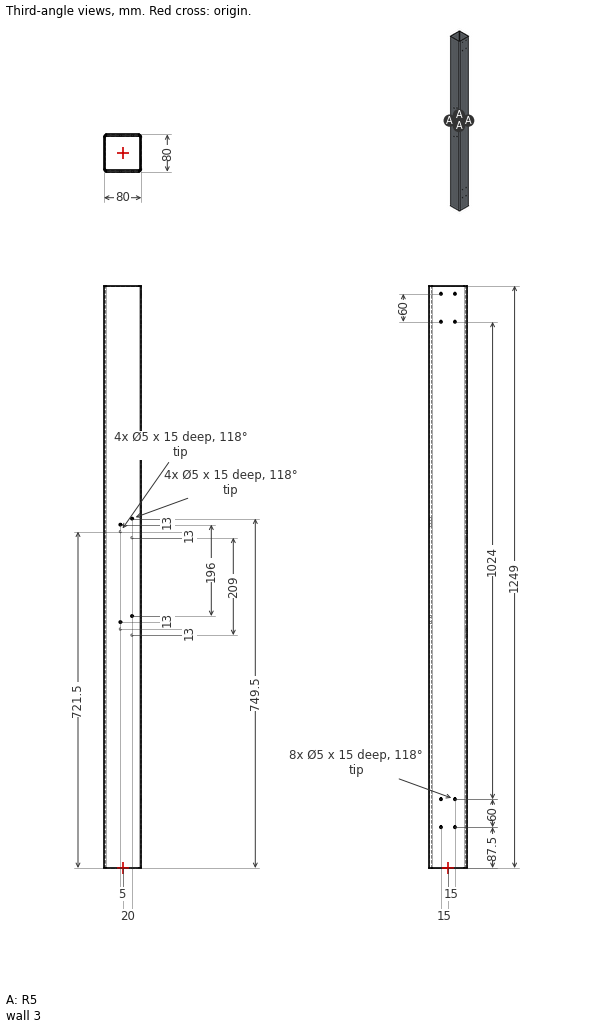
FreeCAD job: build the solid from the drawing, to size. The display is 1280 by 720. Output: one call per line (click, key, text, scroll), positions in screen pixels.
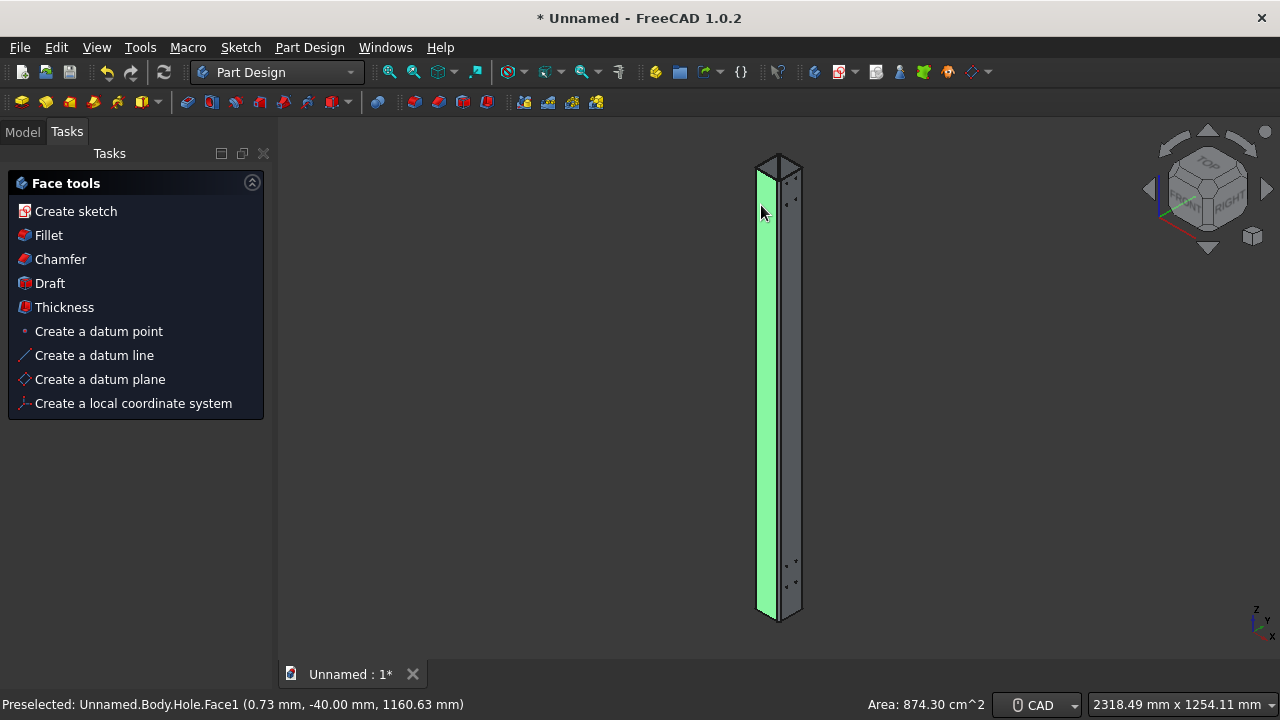
click(840, 72)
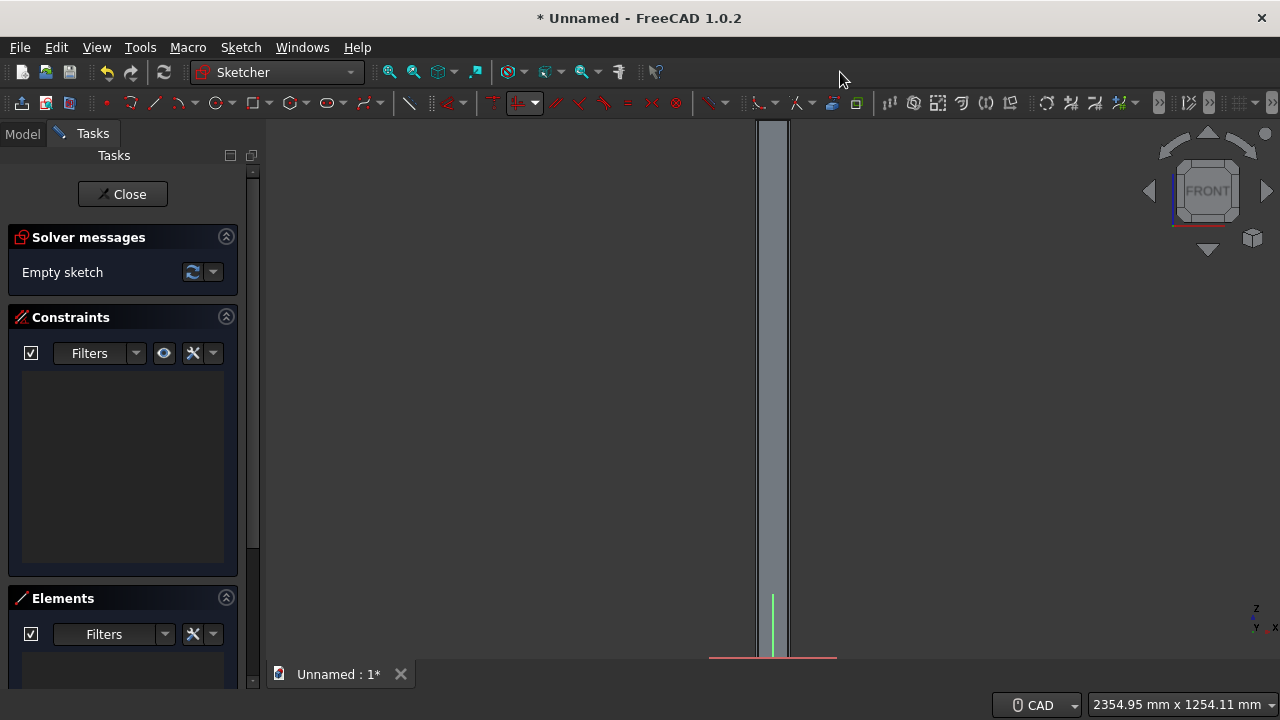
scroll(807, 380, up, 6)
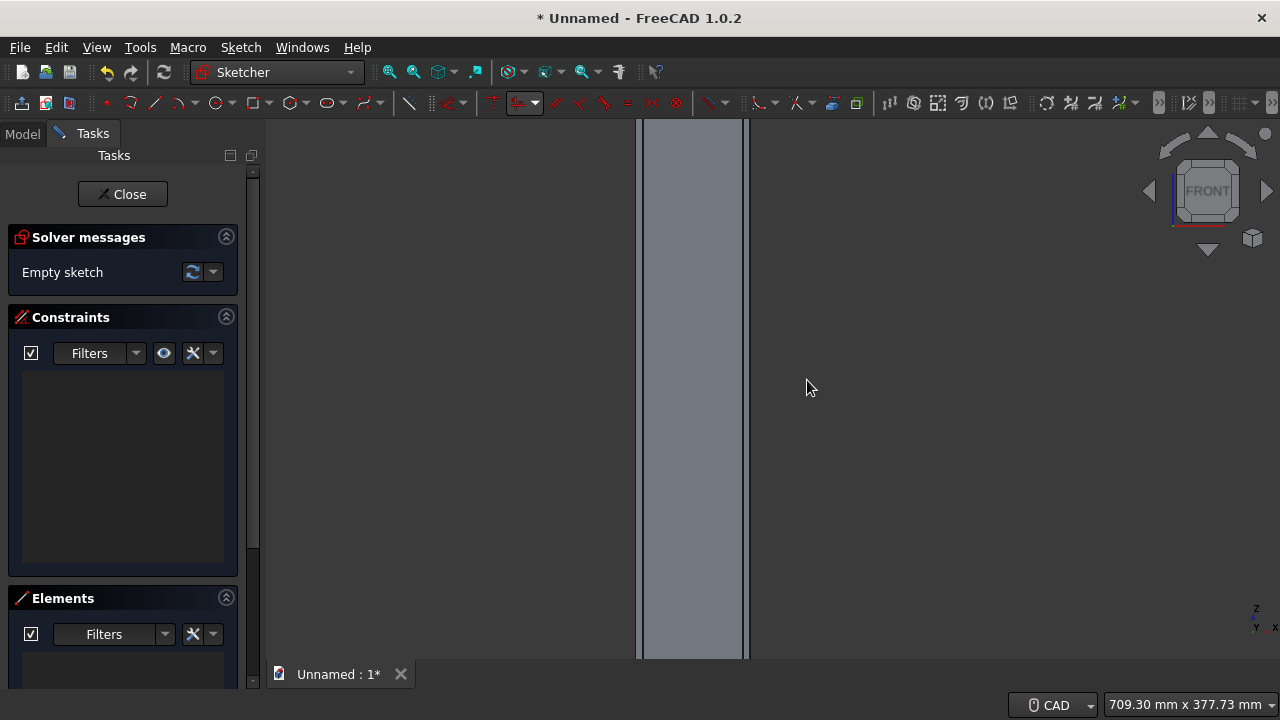
click(216, 104)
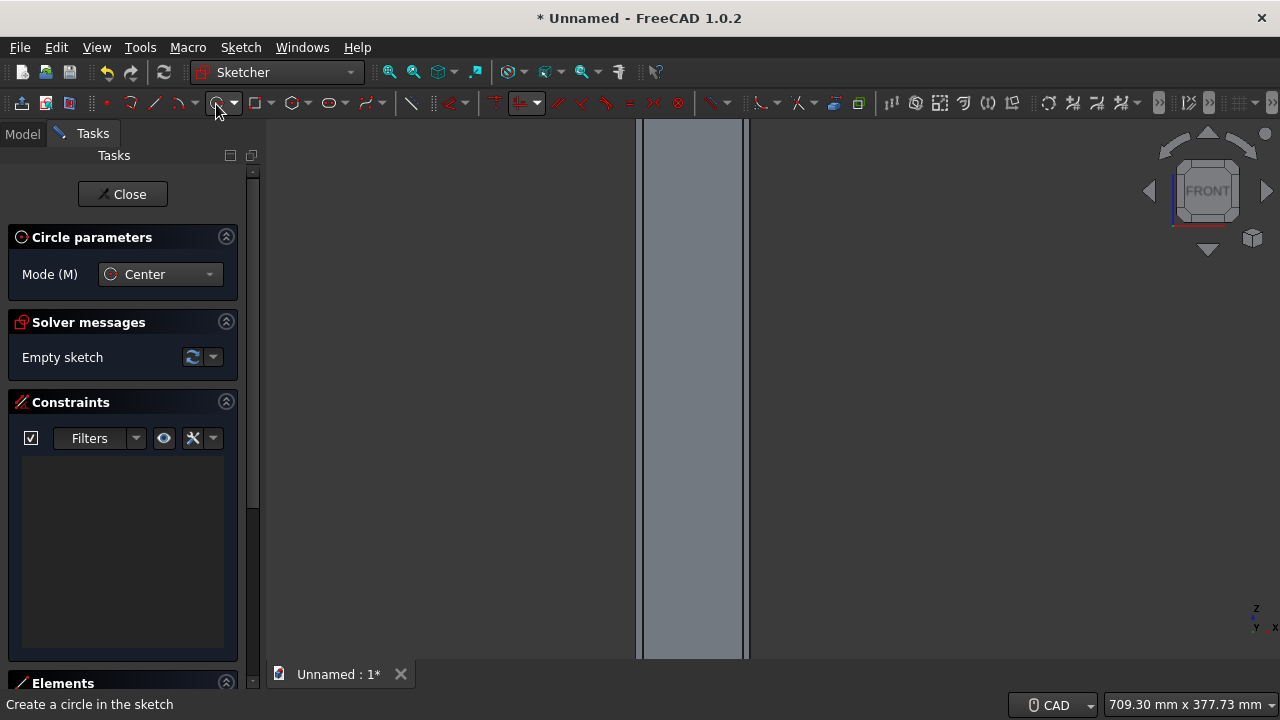
scroll(721, 230, up, 10)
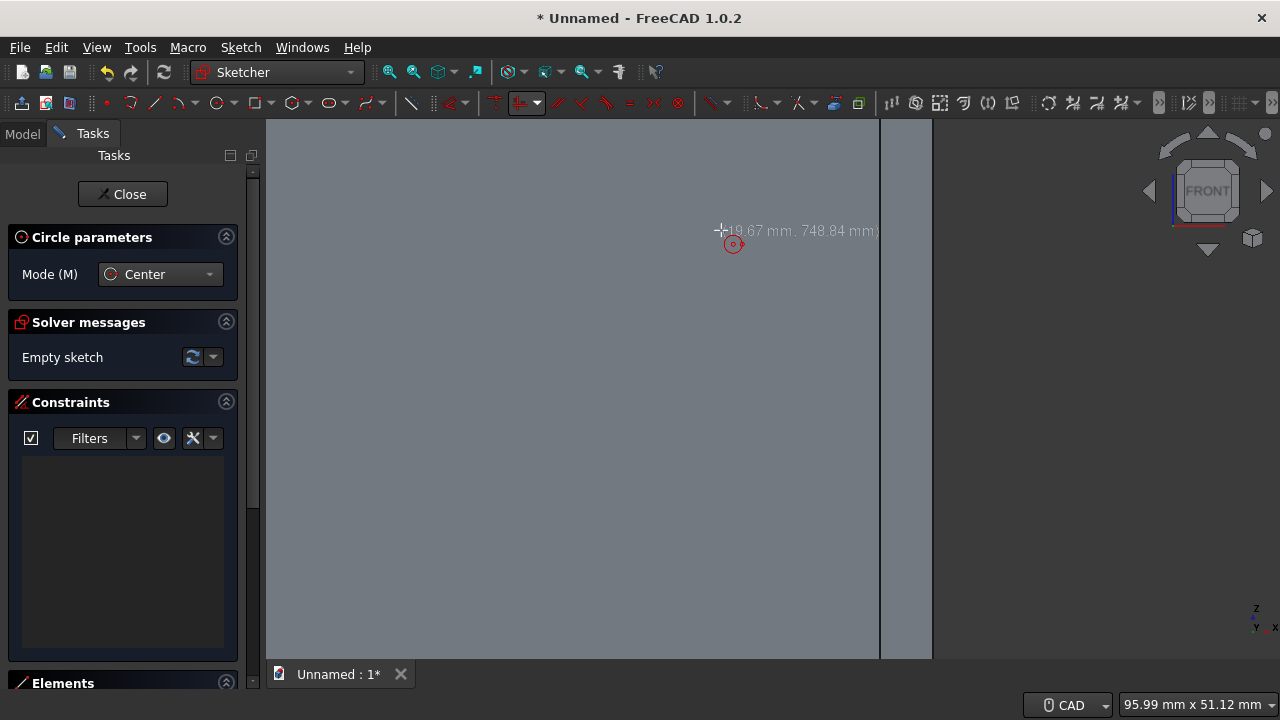
scroll(722, 231, down, 10)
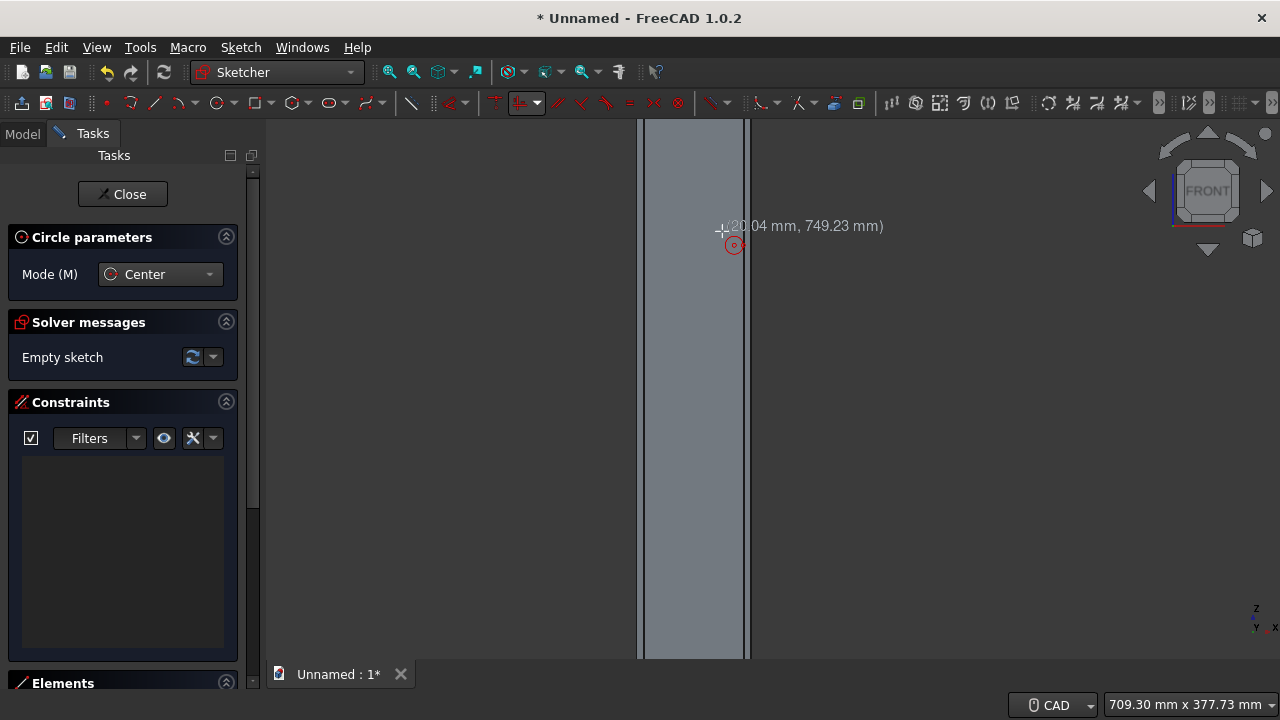
click(722, 231)
move(725, 228)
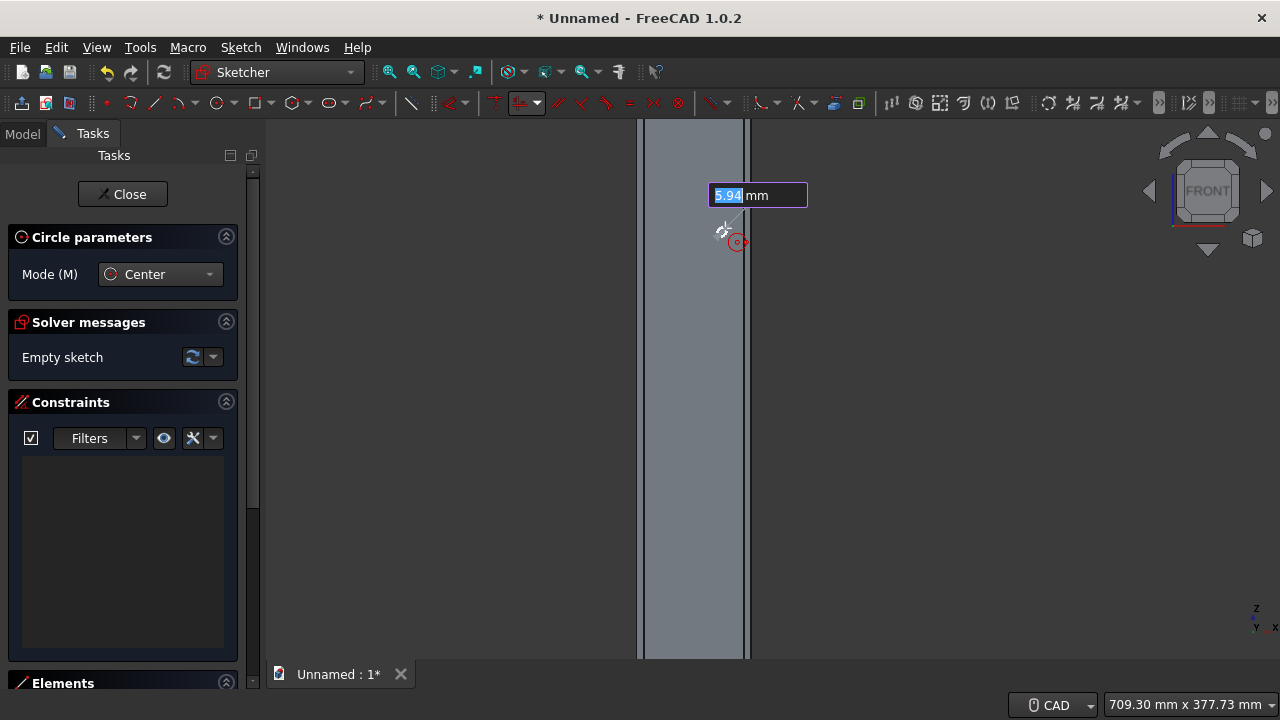
text(5)
key(Return)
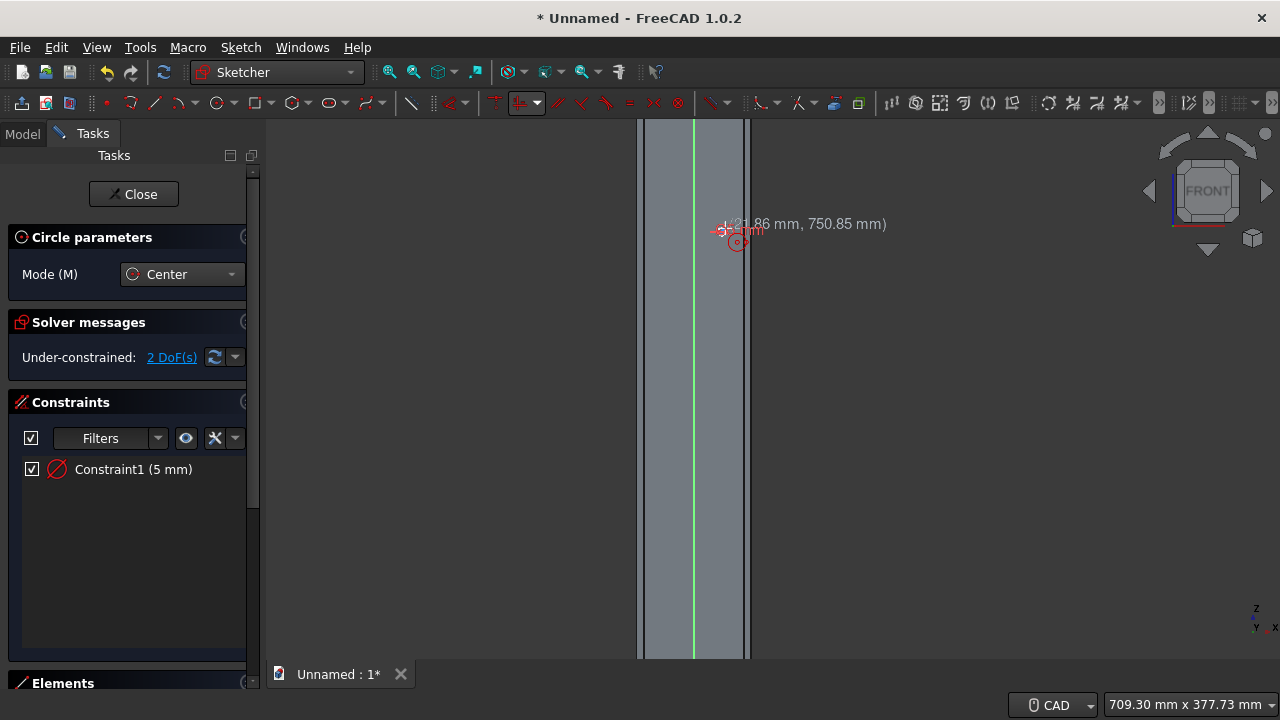
scroll(687, 250, up, 10)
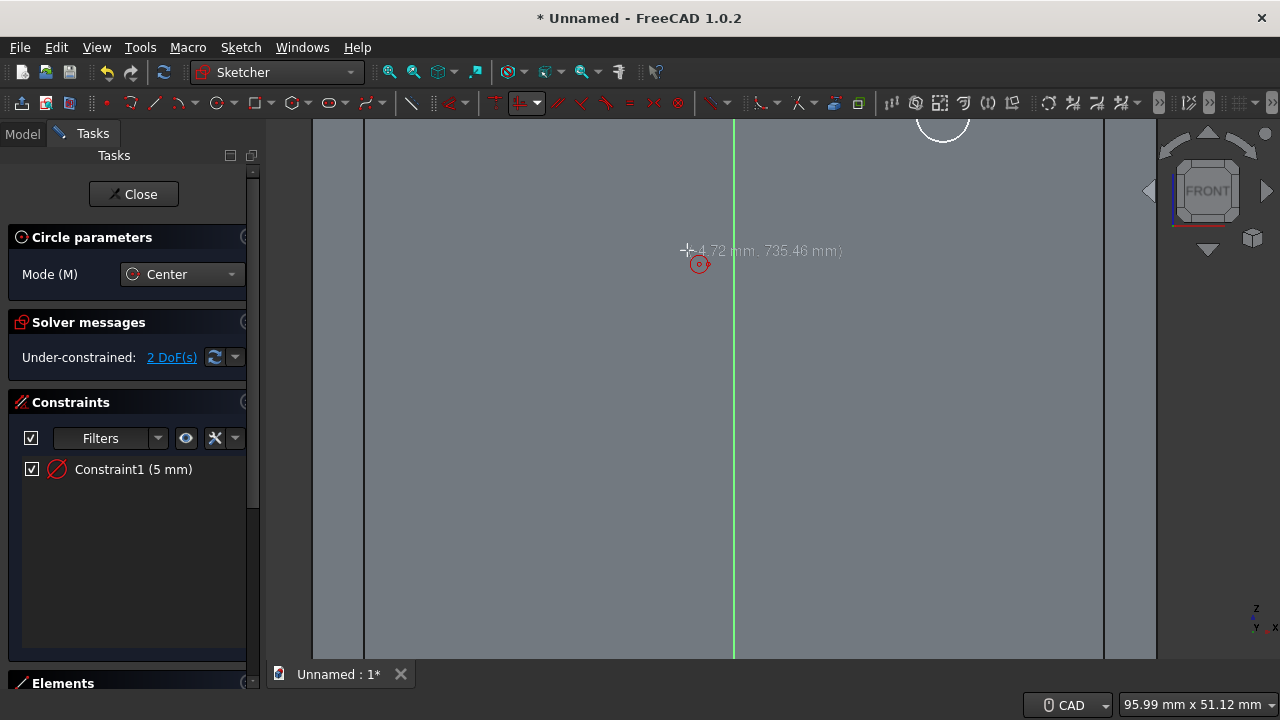
scroll(687, 250, down, 10)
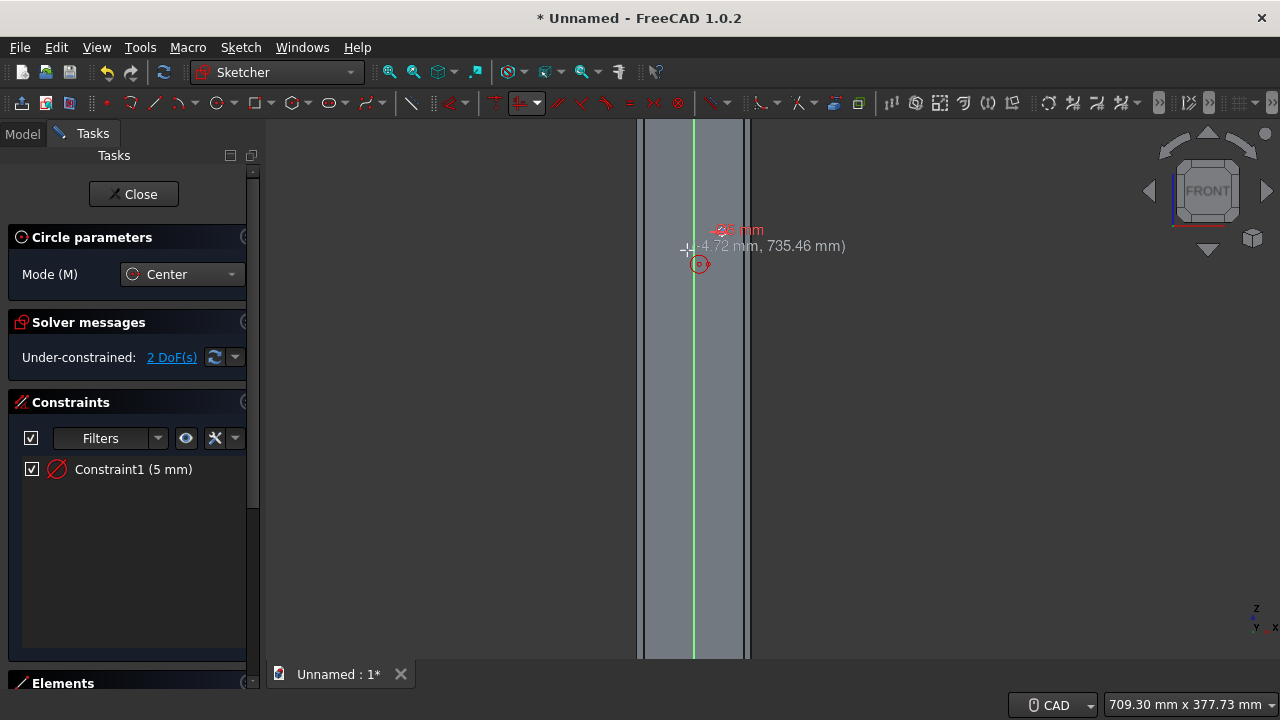
scroll(687, 250, up, 4)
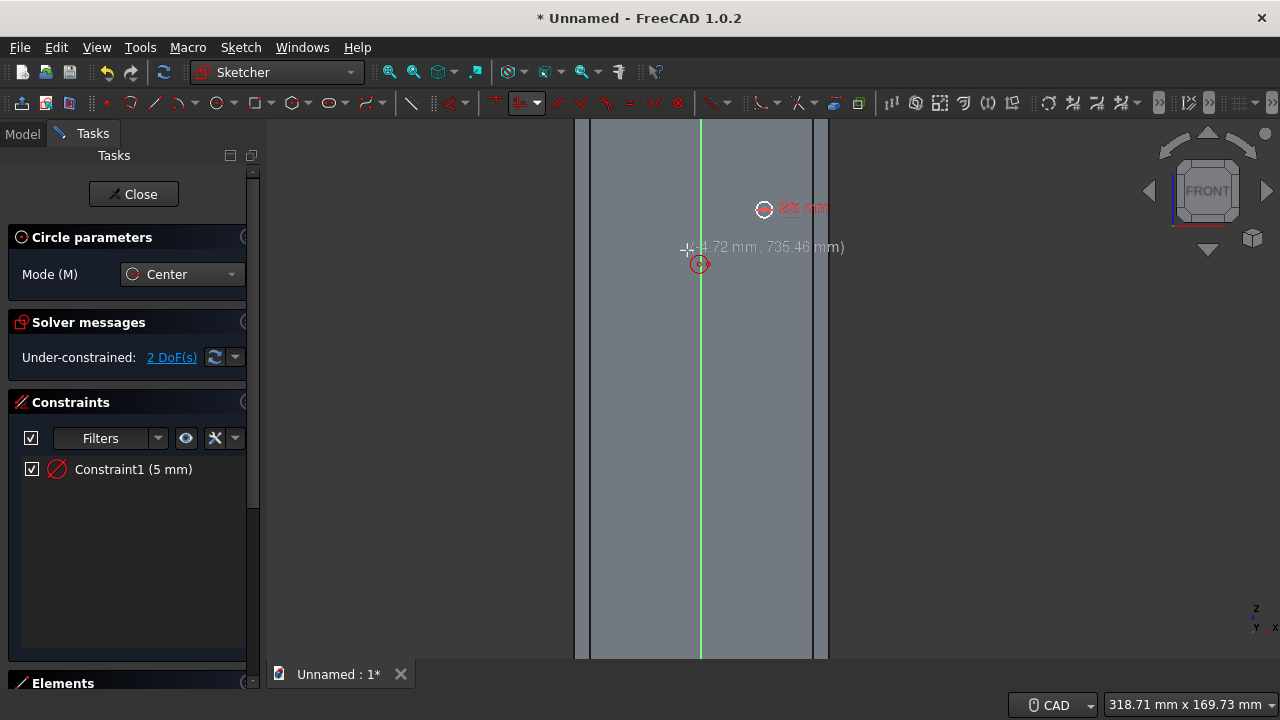
click(686, 249)
move(680, 243)